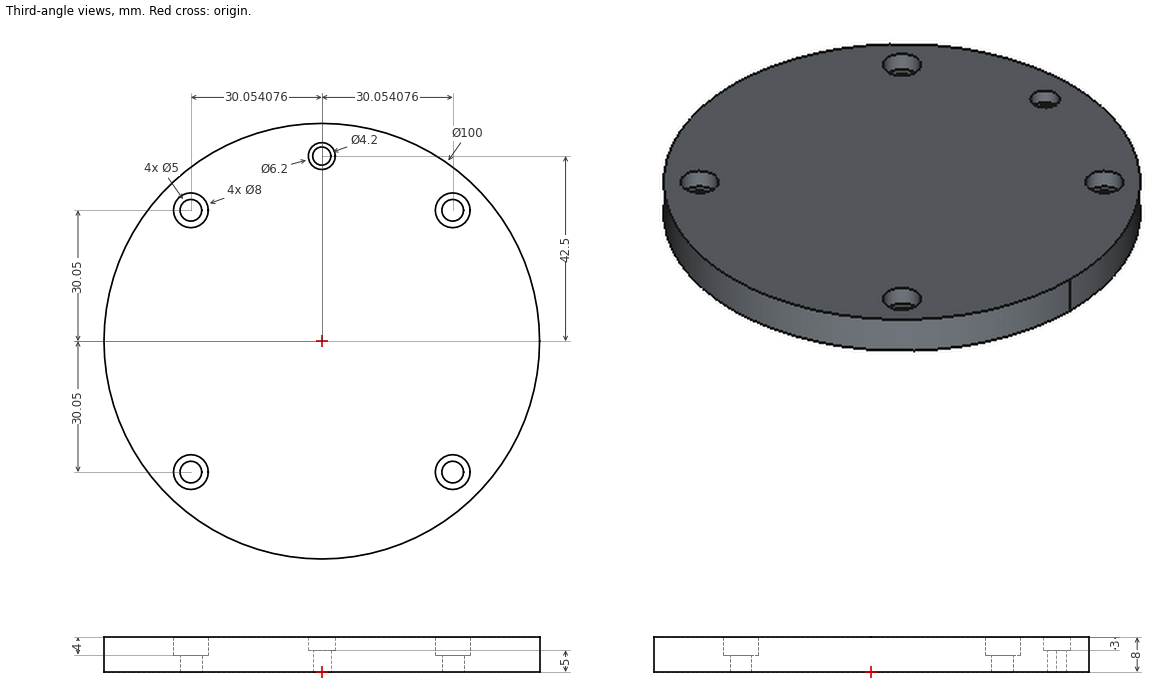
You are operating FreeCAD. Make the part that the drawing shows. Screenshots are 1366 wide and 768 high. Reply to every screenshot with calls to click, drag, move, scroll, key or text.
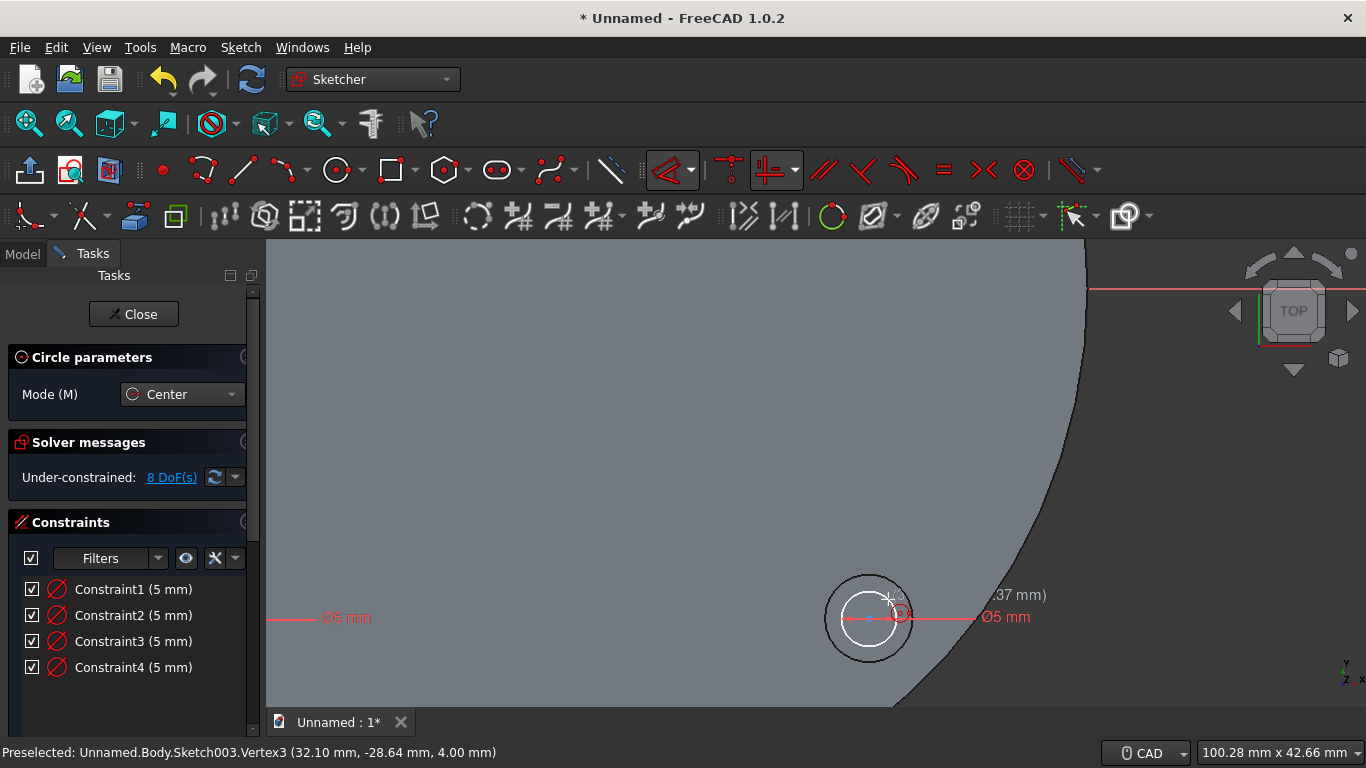
scroll(869, 619, down, 5)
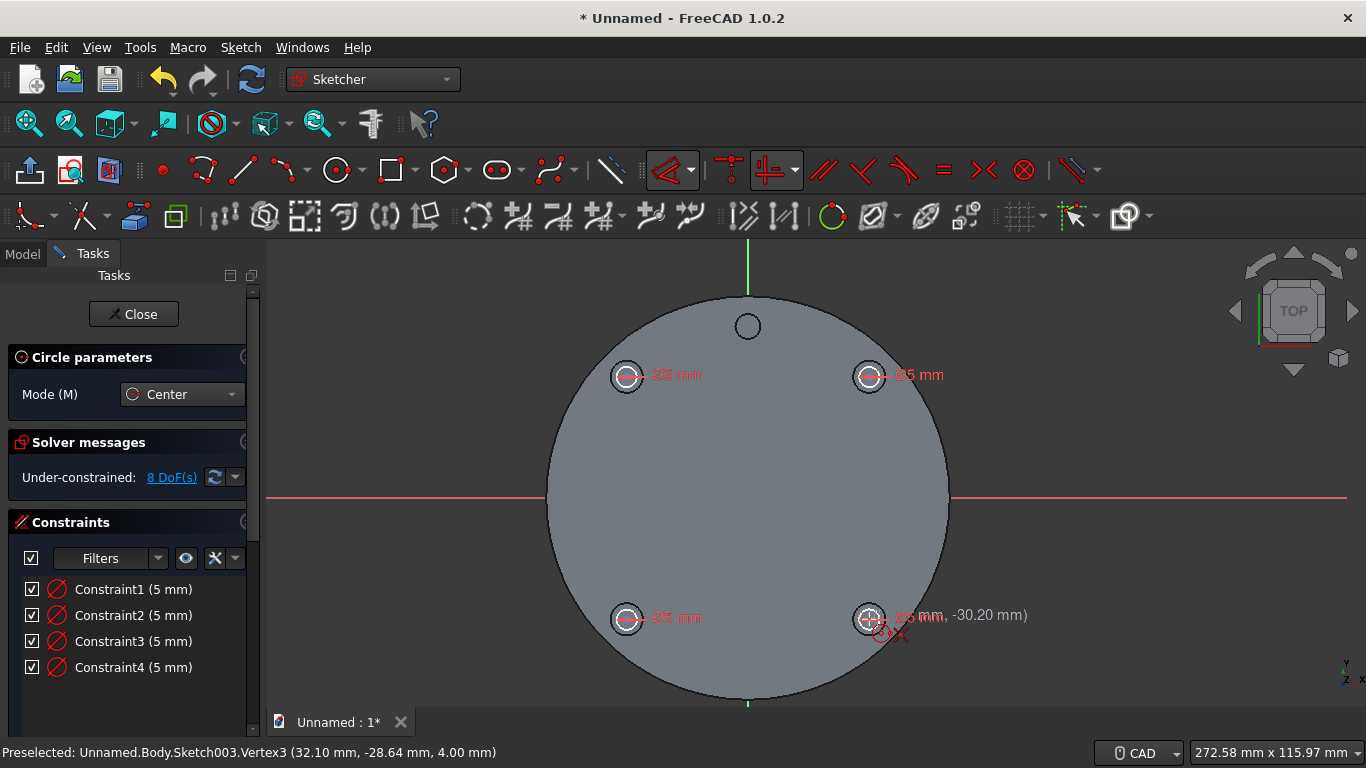
scroll(748, 327, up, 5)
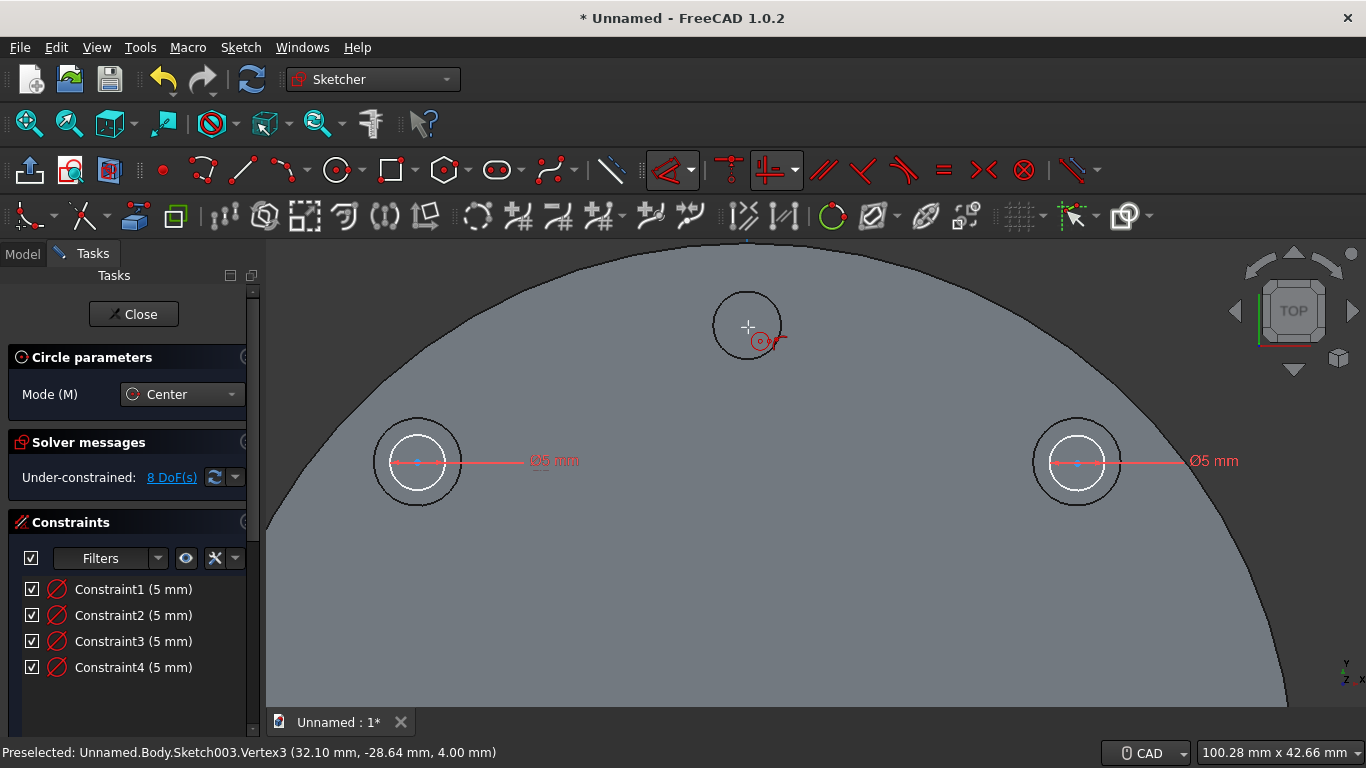
click(747, 325)
move(763, 309)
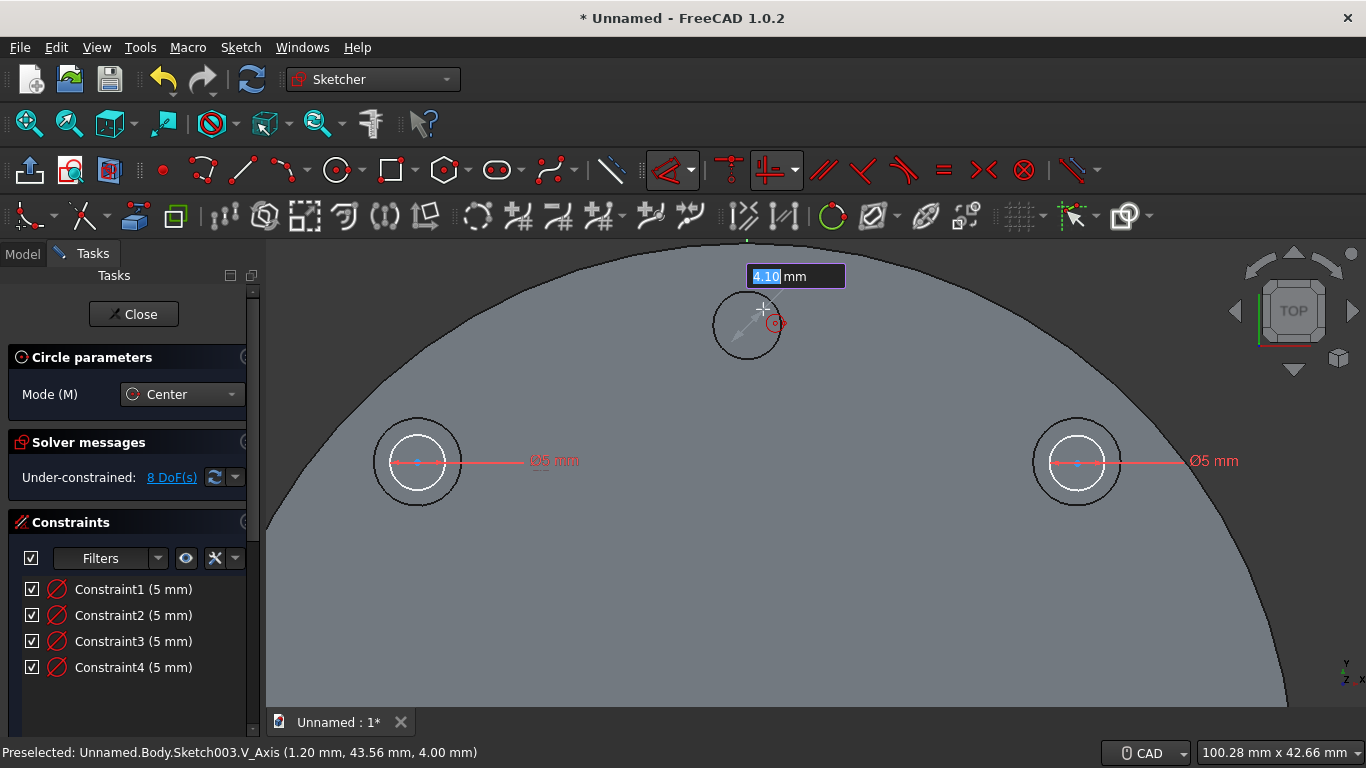
text(4.2)
key(Return)
key(Escape)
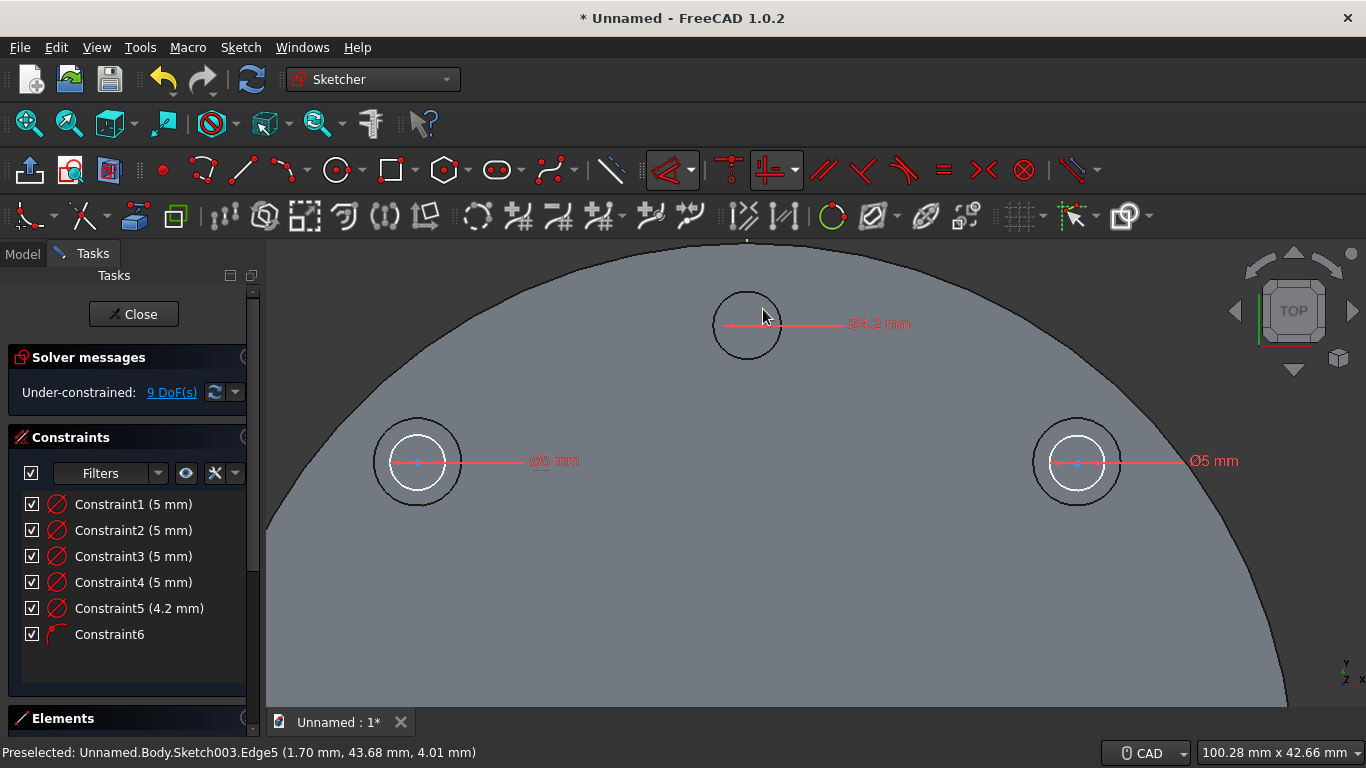
click(417, 463)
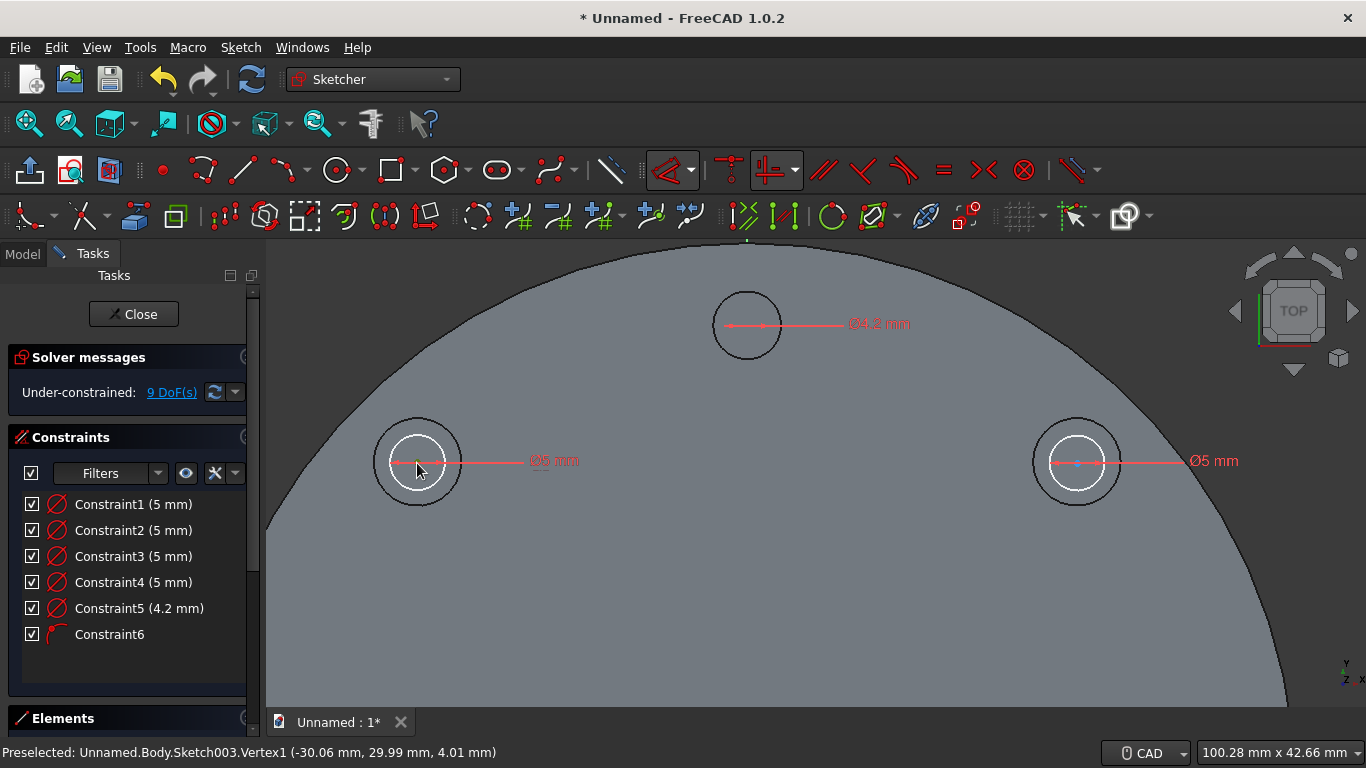
click(1077, 463)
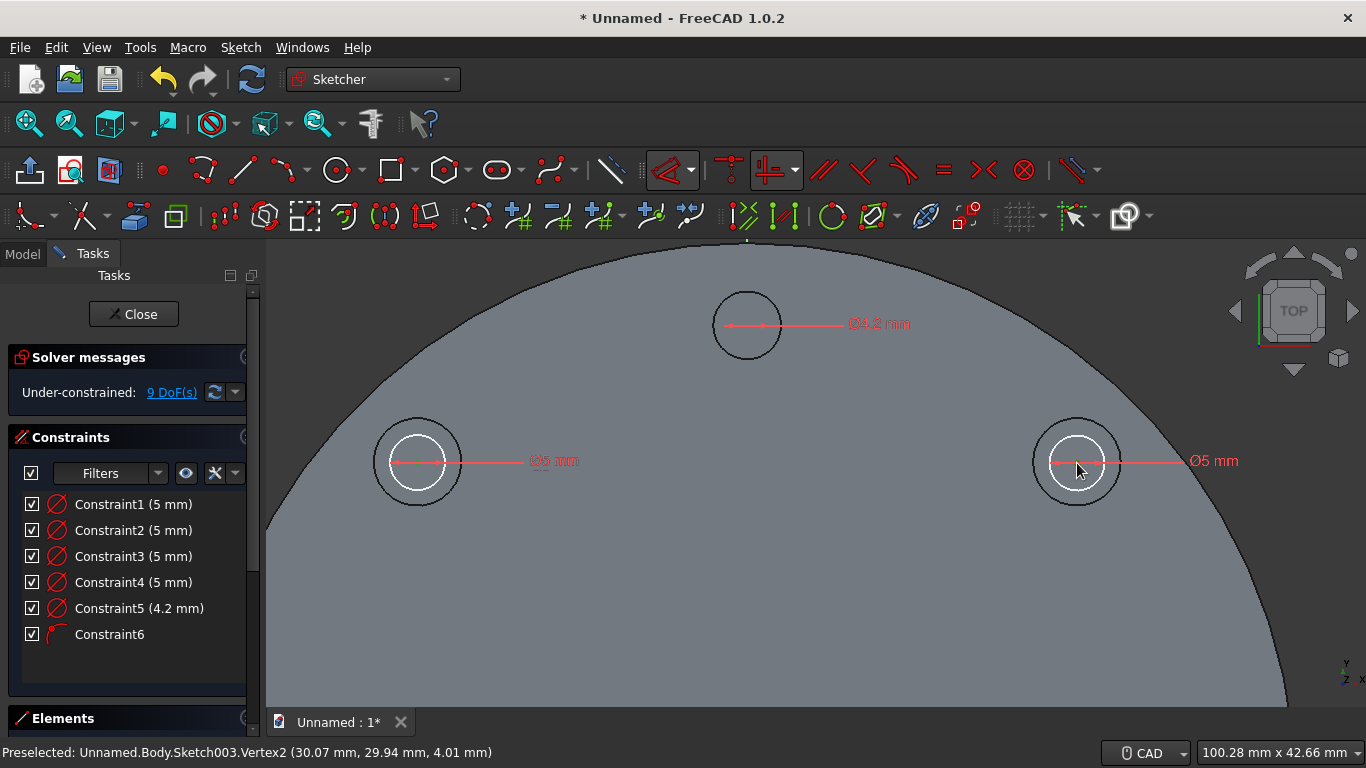
key(h)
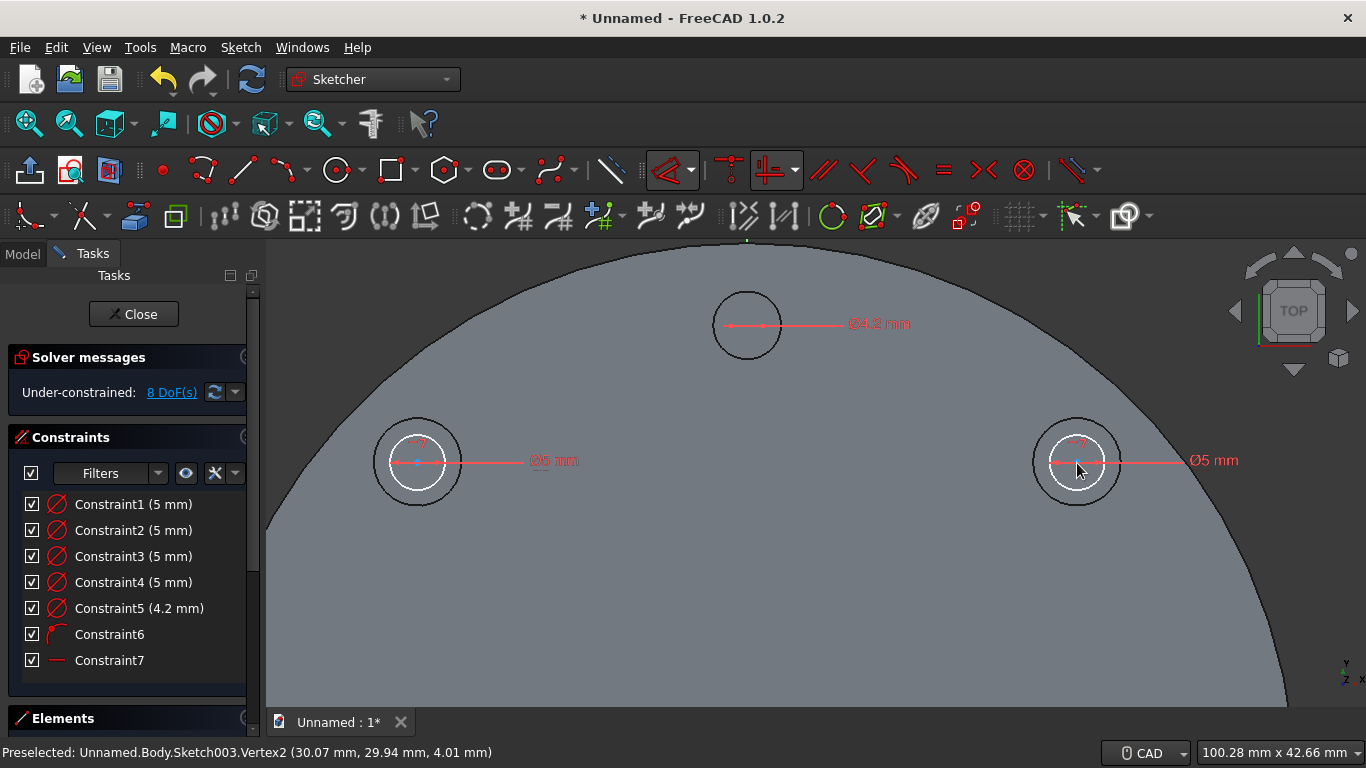
click(417, 463)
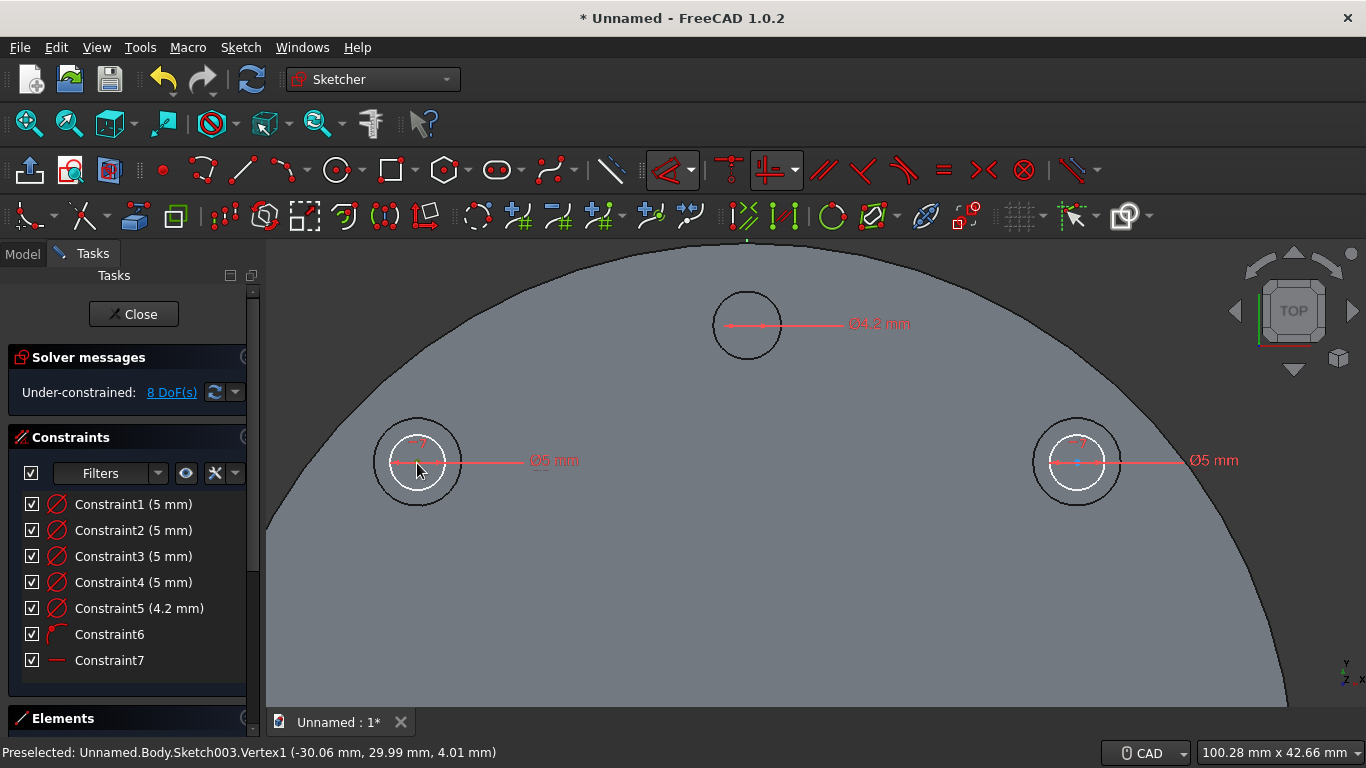
scroll(748, 326, down, 5)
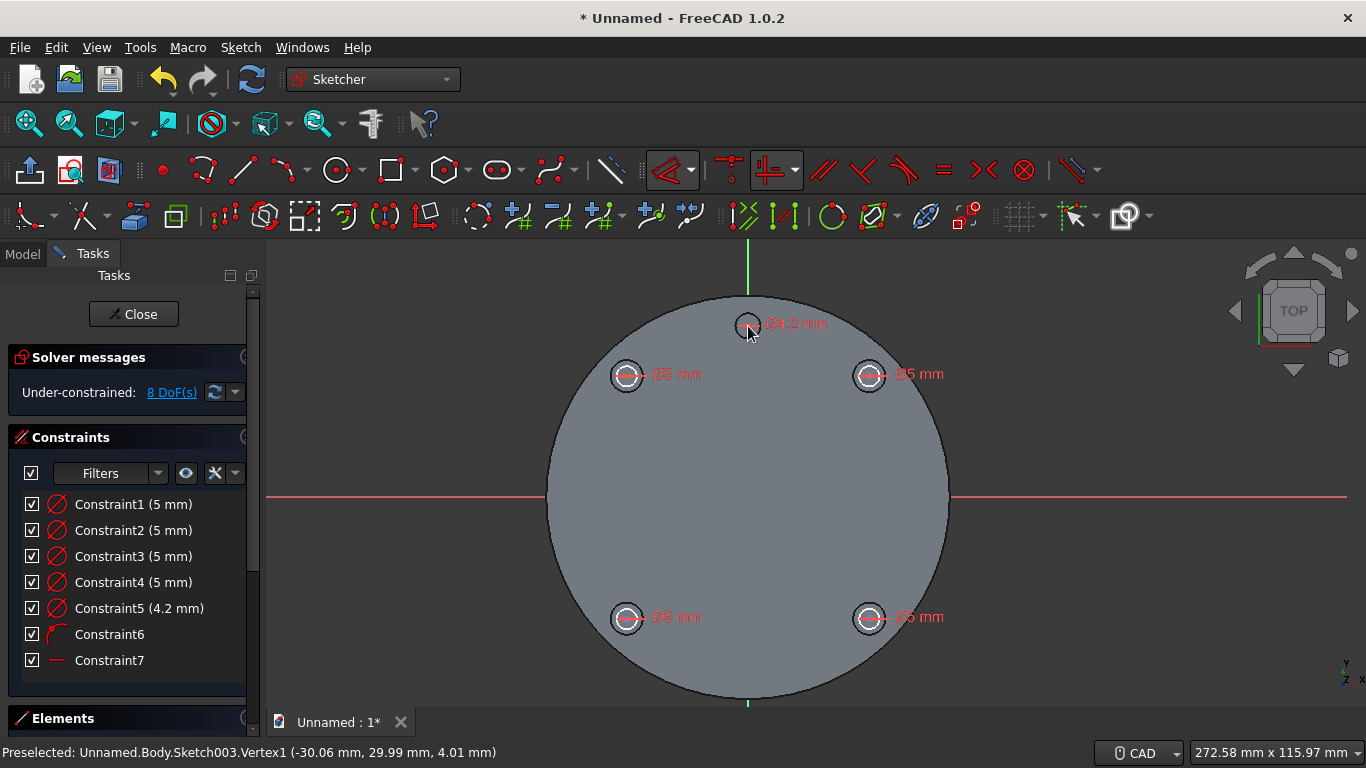
click(627, 619)